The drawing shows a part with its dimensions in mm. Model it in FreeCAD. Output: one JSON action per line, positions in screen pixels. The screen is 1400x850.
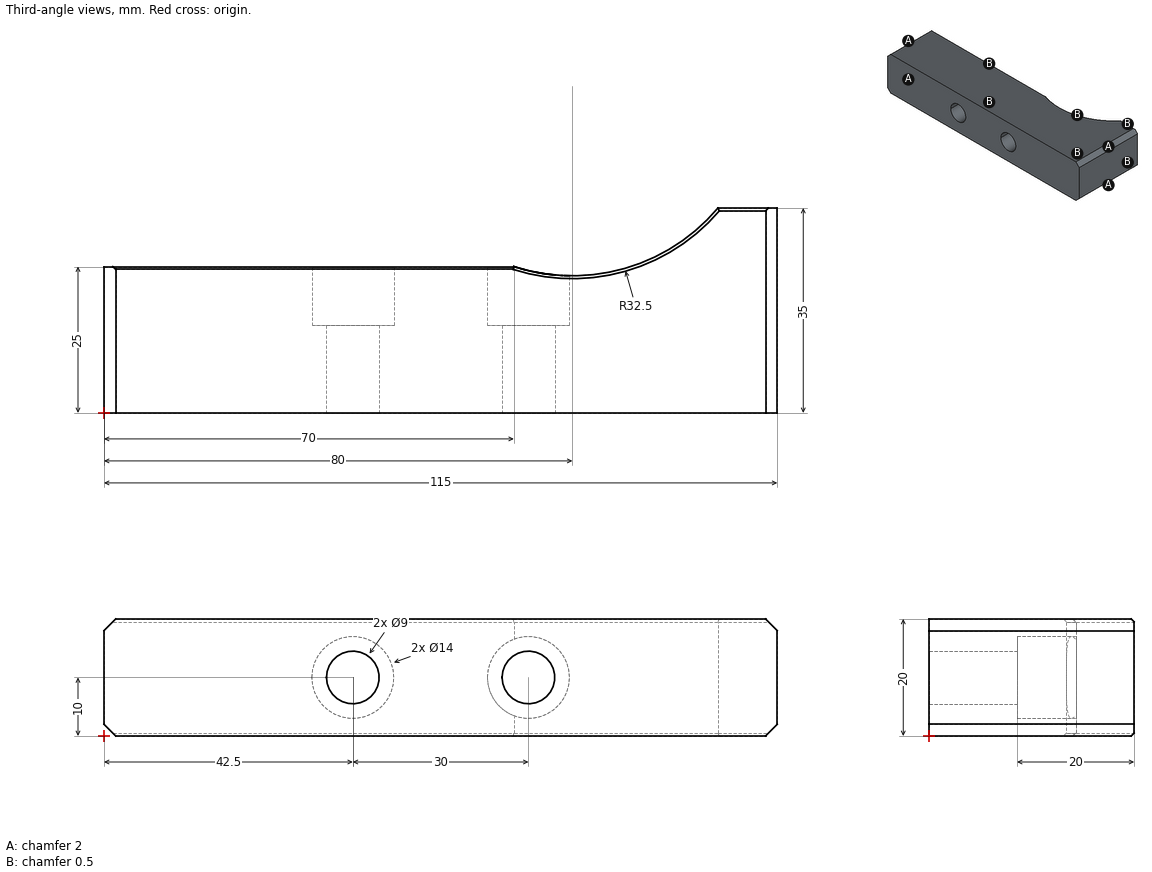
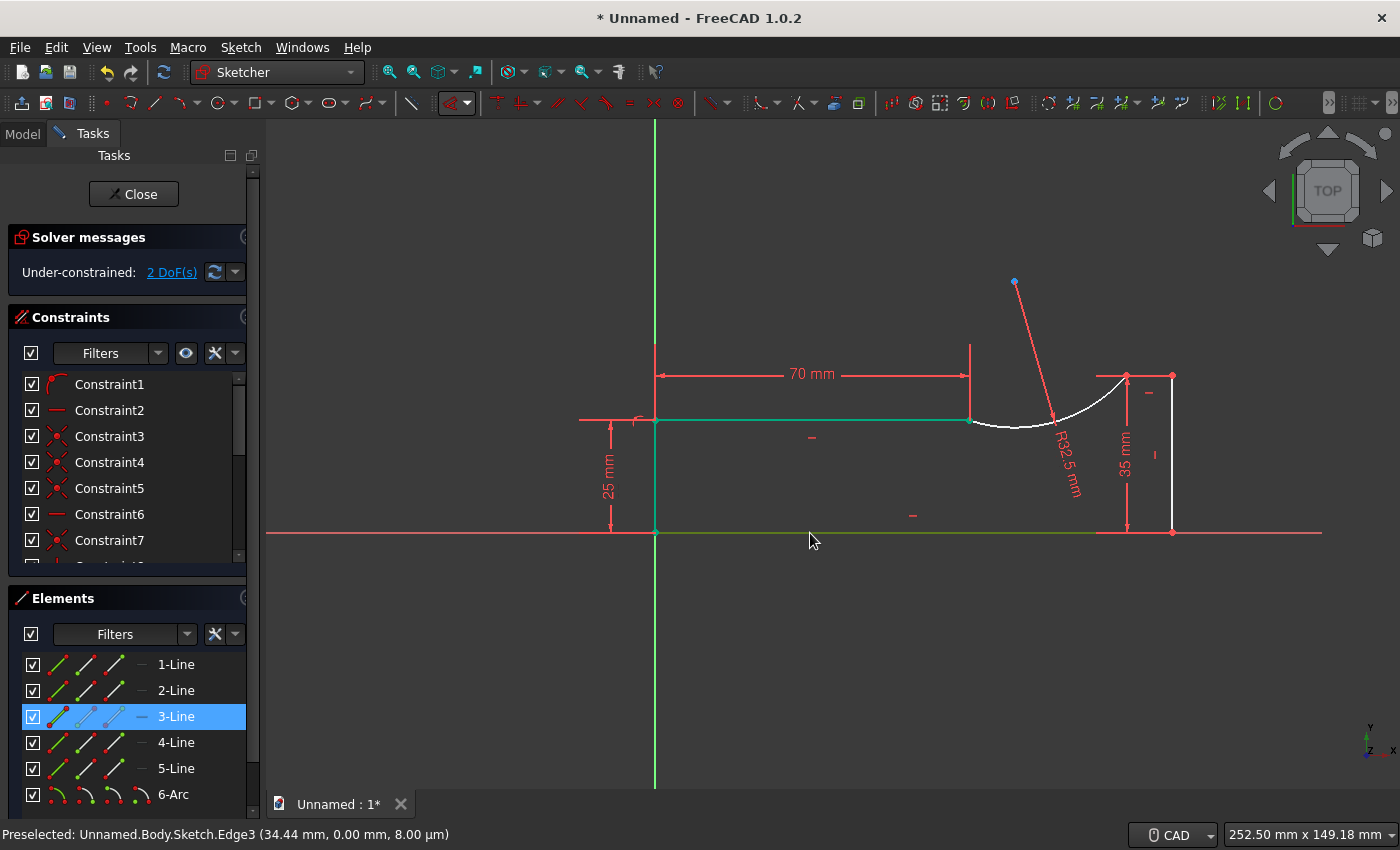
{"action": "left_click", "coordinate": [470, 104]}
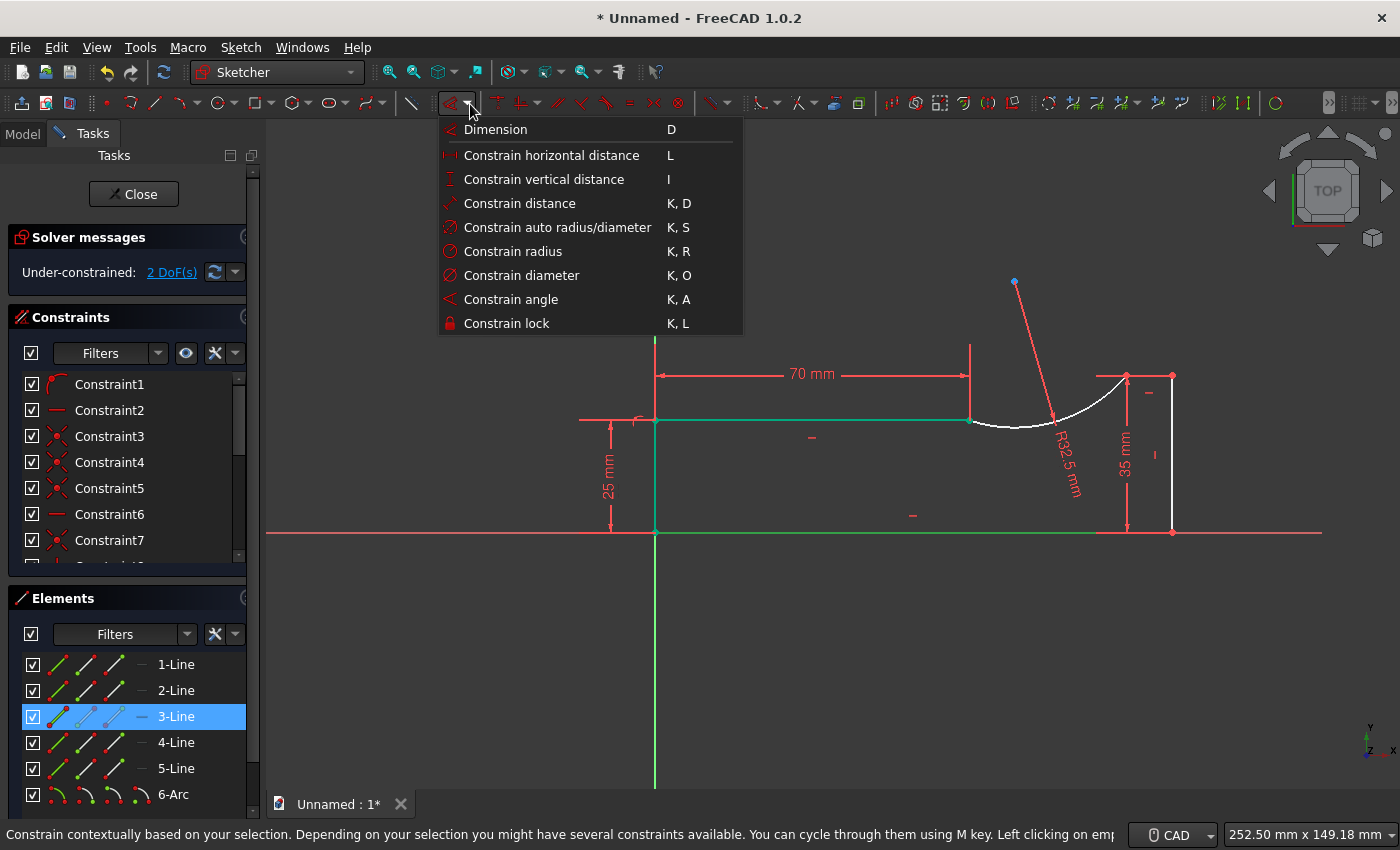
{"action": "left_click", "coordinate": [591, 155]}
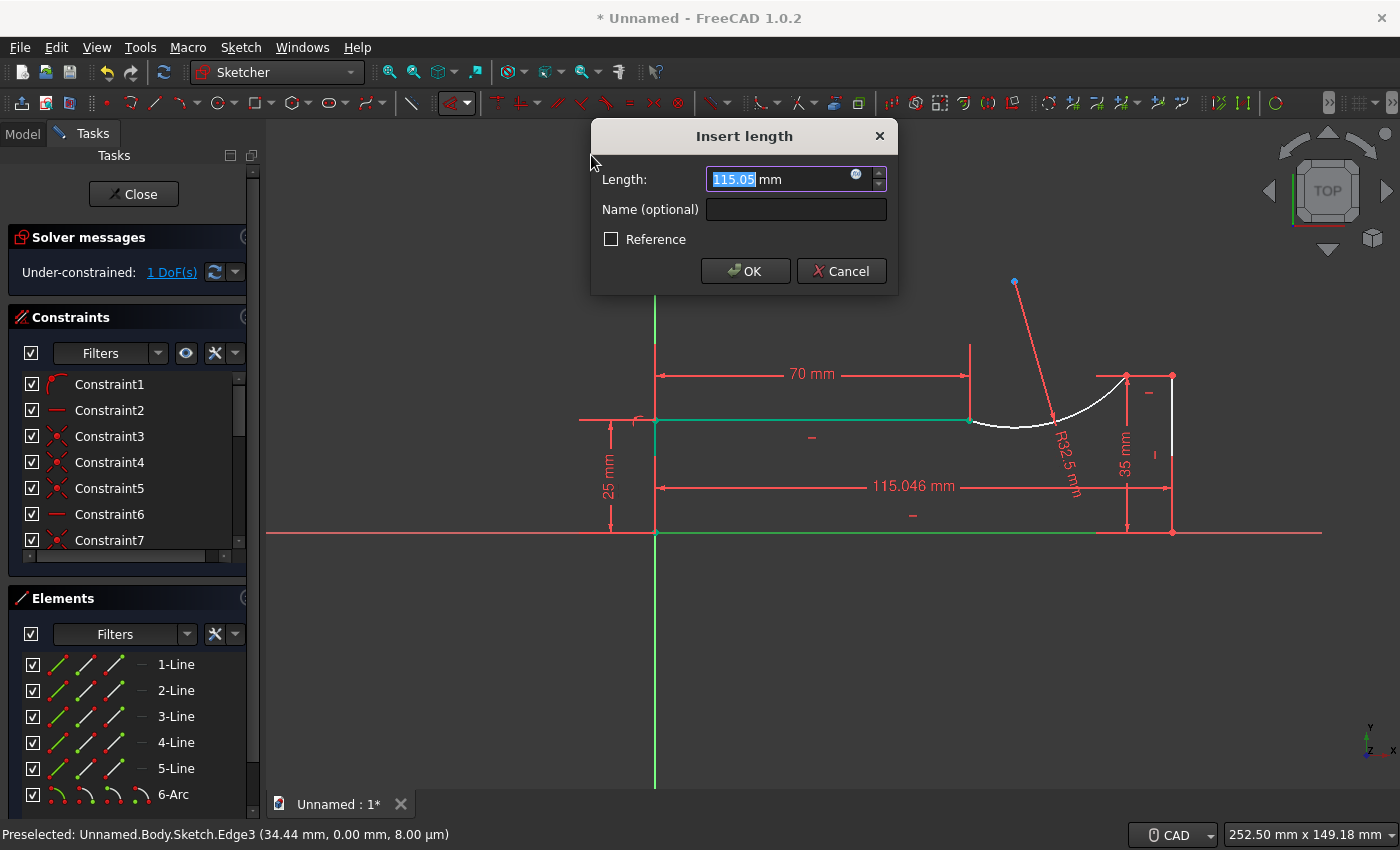
{"action": "type", "text": "115"}
{"action": "key", "text": "Return"}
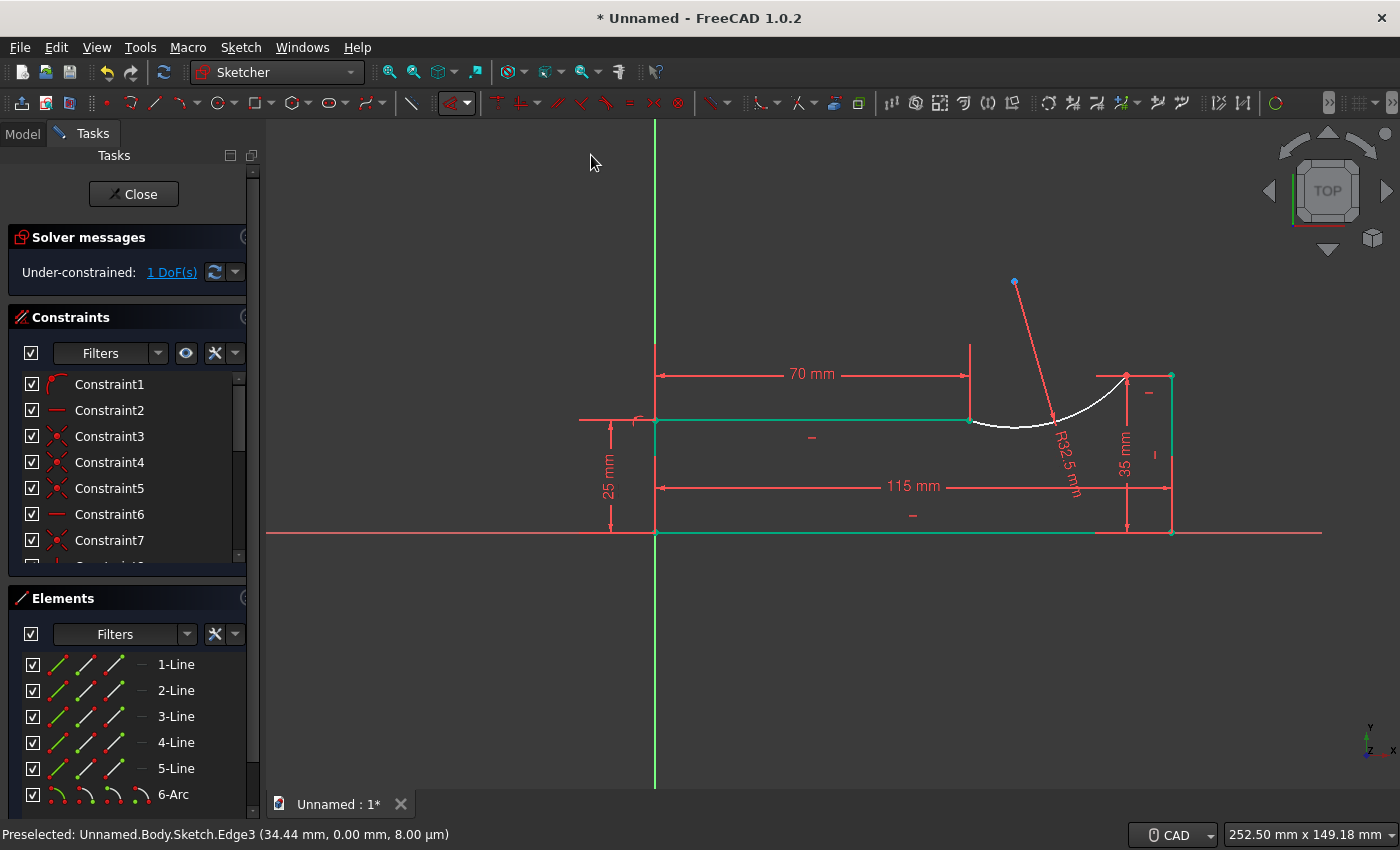
{"action": "left_click", "coordinate": [1015, 282]}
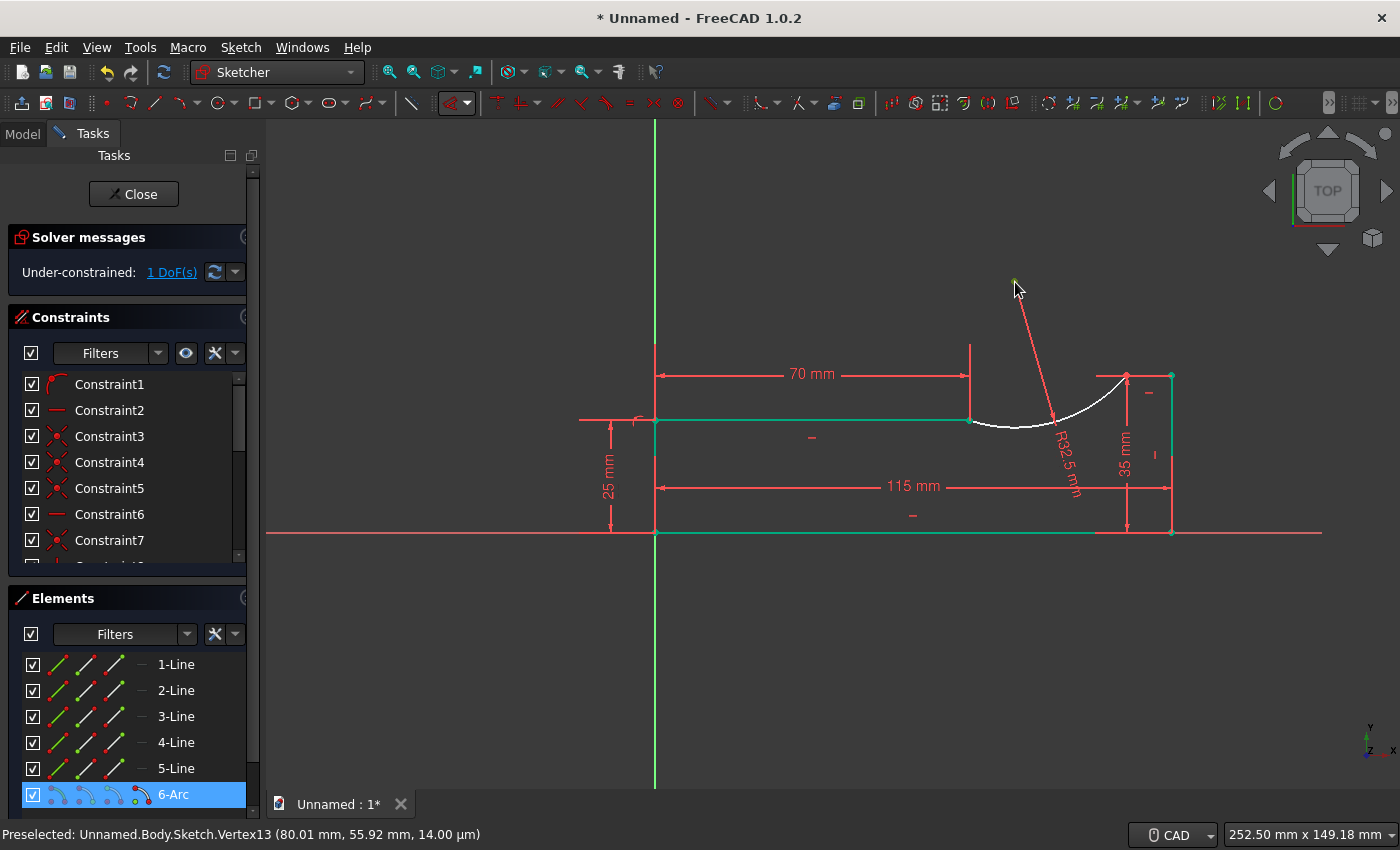
{"action": "key", "text": "l"}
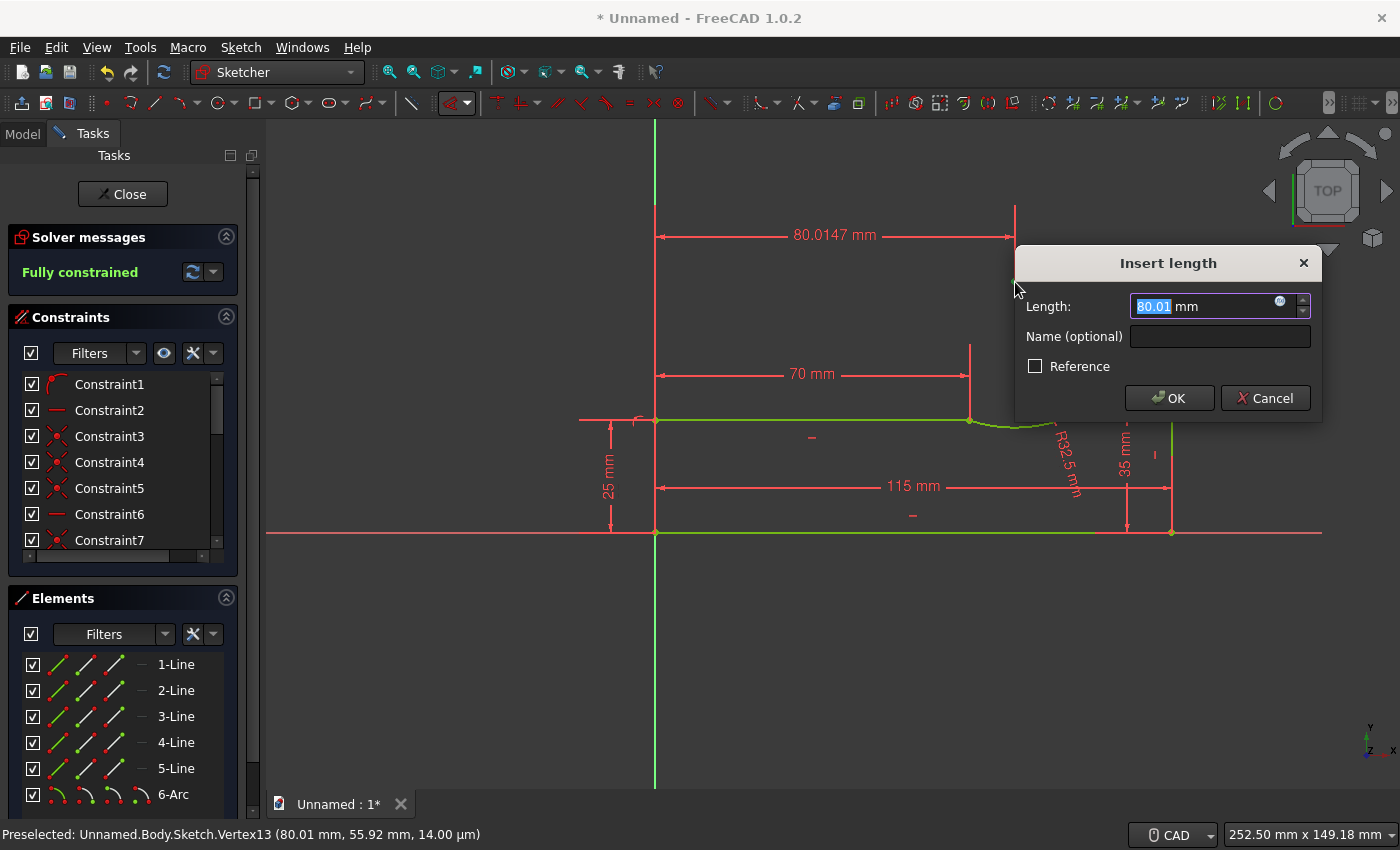
{"action": "type", "text": "80"}
{"action": "key", "text": "Return"}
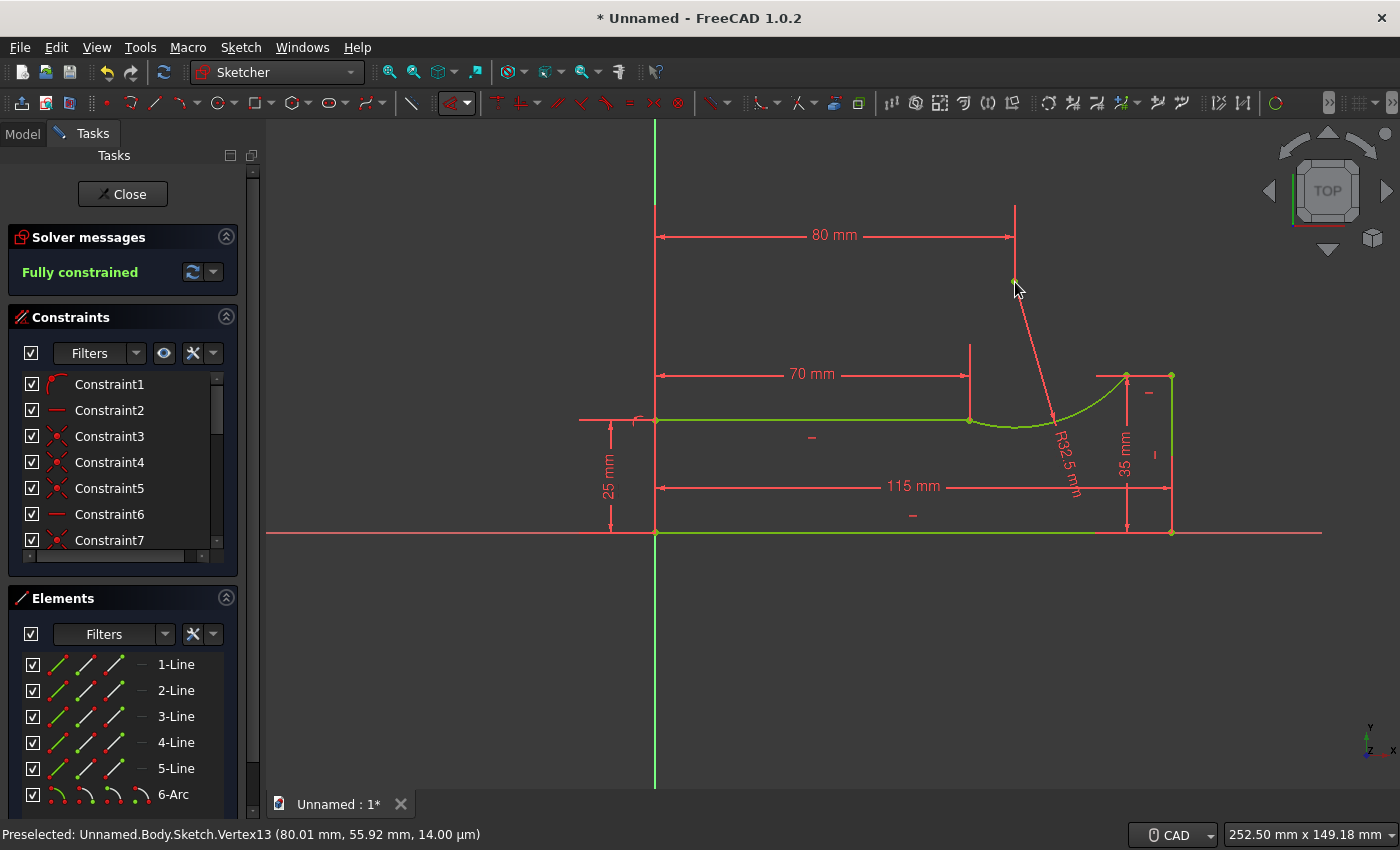
{"action": "left_click", "coordinate": [123, 194]}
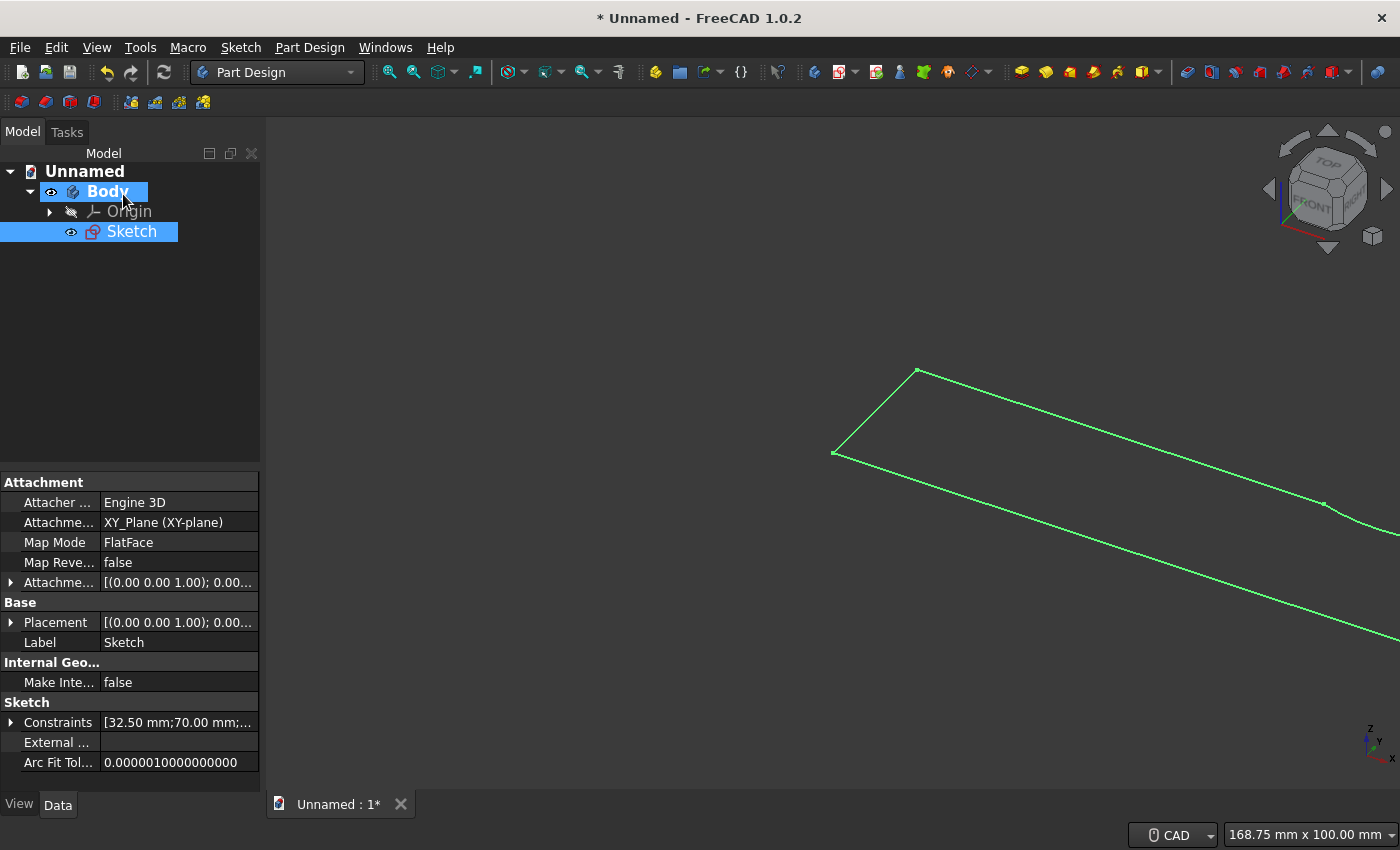
{"action": "left_click", "coordinate": [1022, 72]}